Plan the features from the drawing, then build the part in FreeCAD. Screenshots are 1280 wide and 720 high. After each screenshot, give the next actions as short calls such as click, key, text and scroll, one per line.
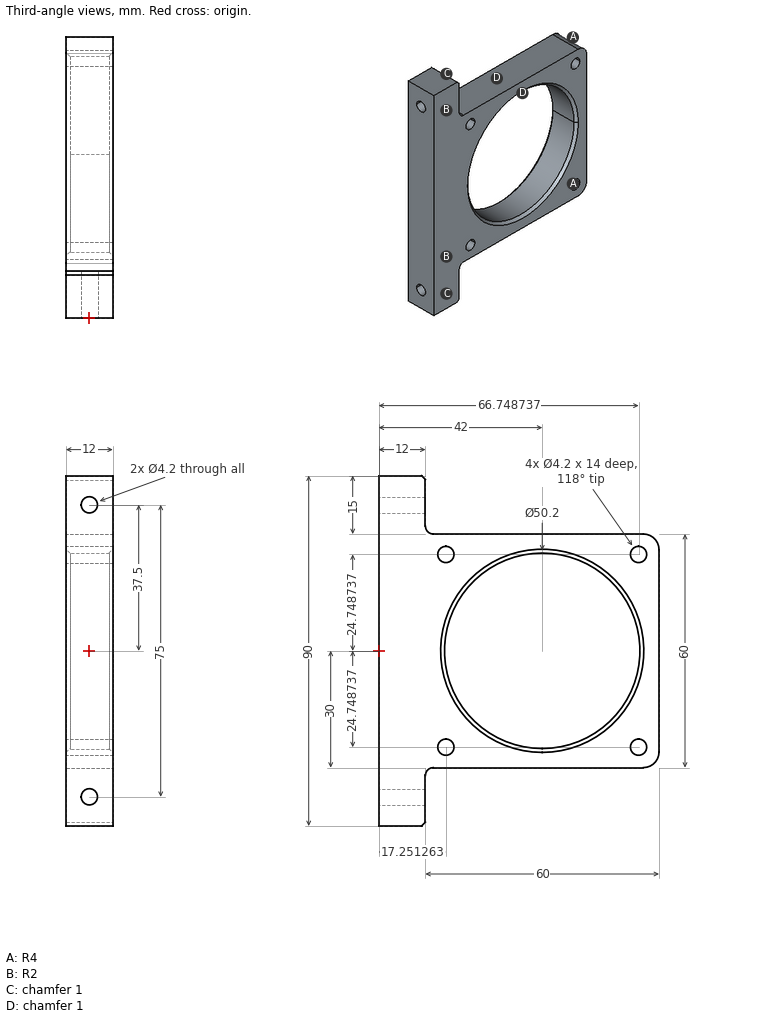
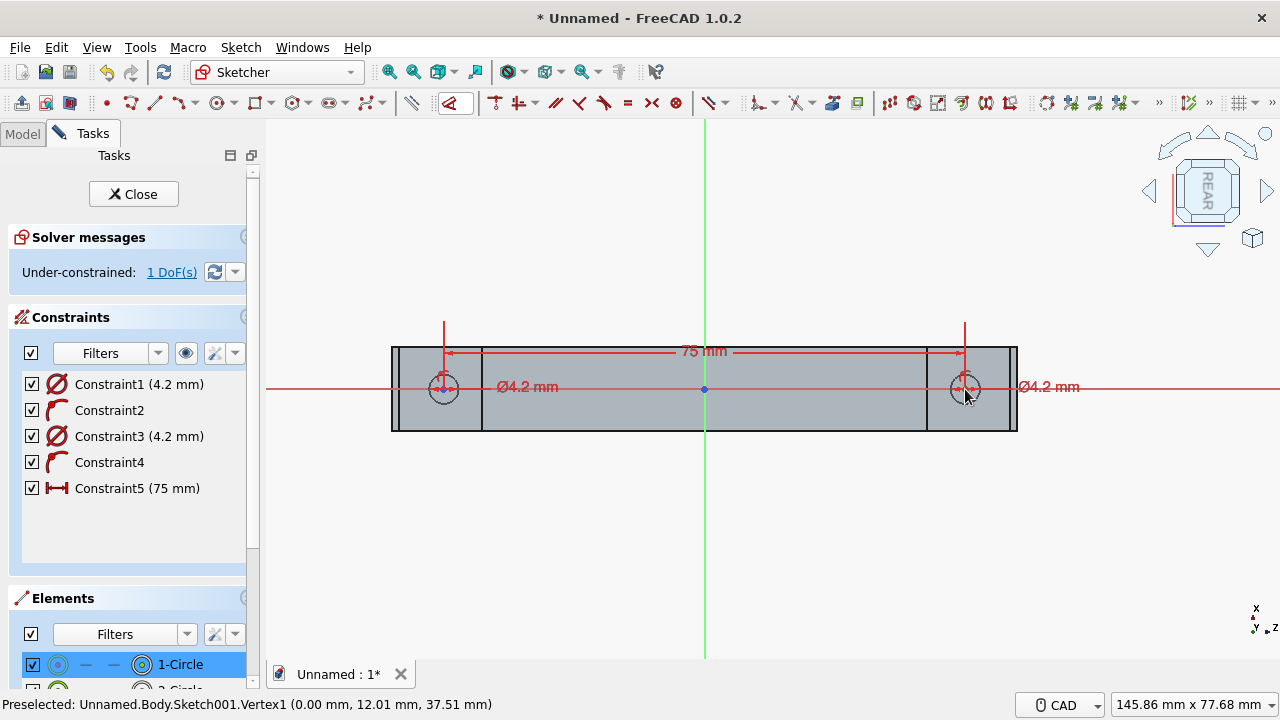
key(l)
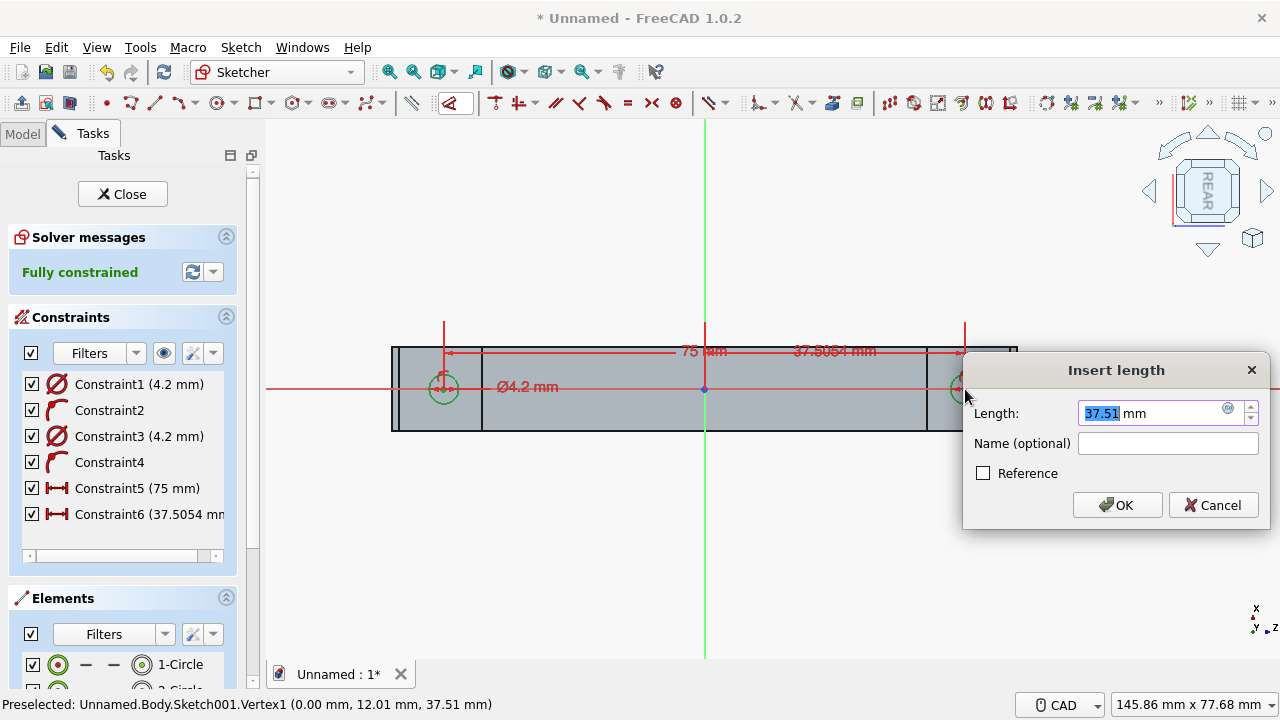
text(37.5)
key(Return)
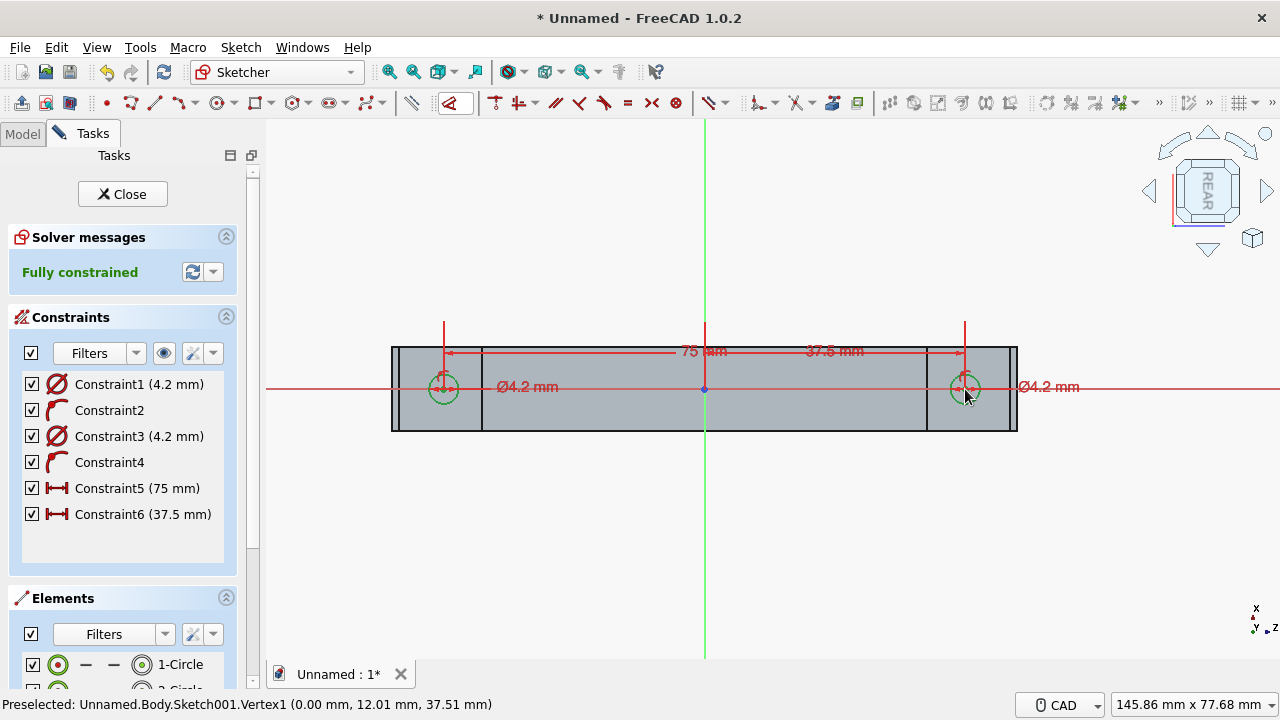
click(123, 194)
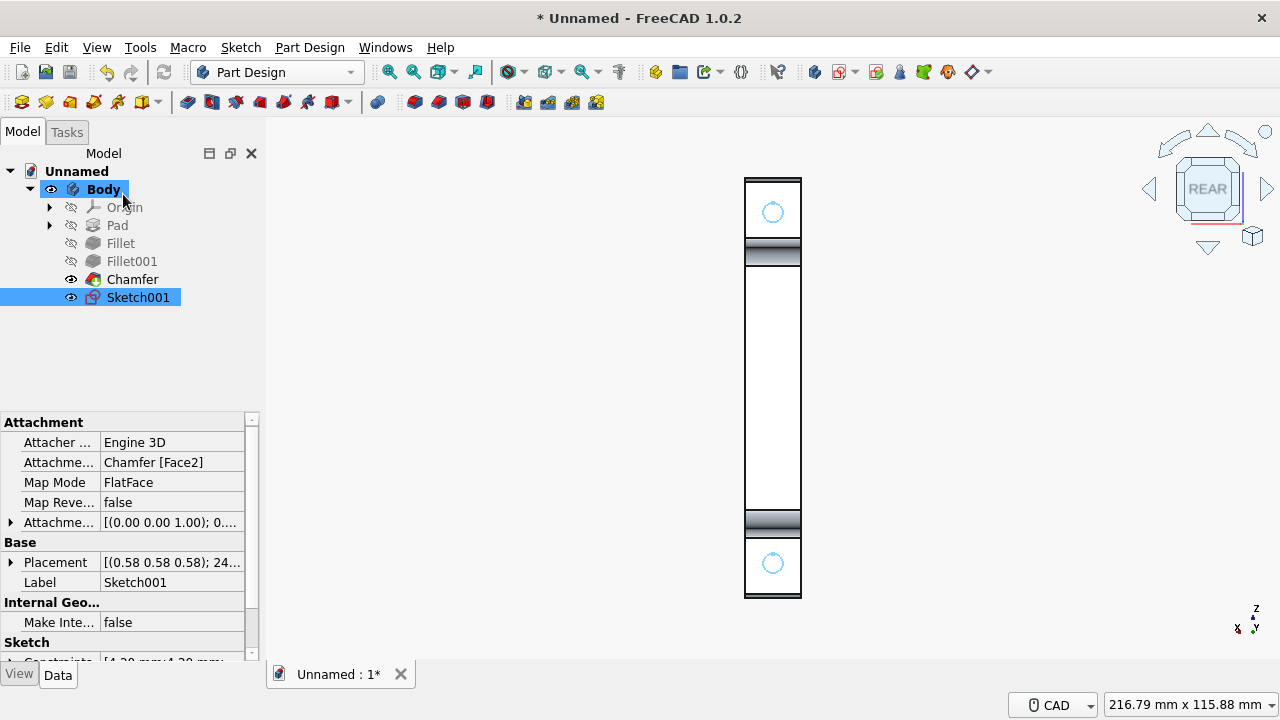
click(212, 102)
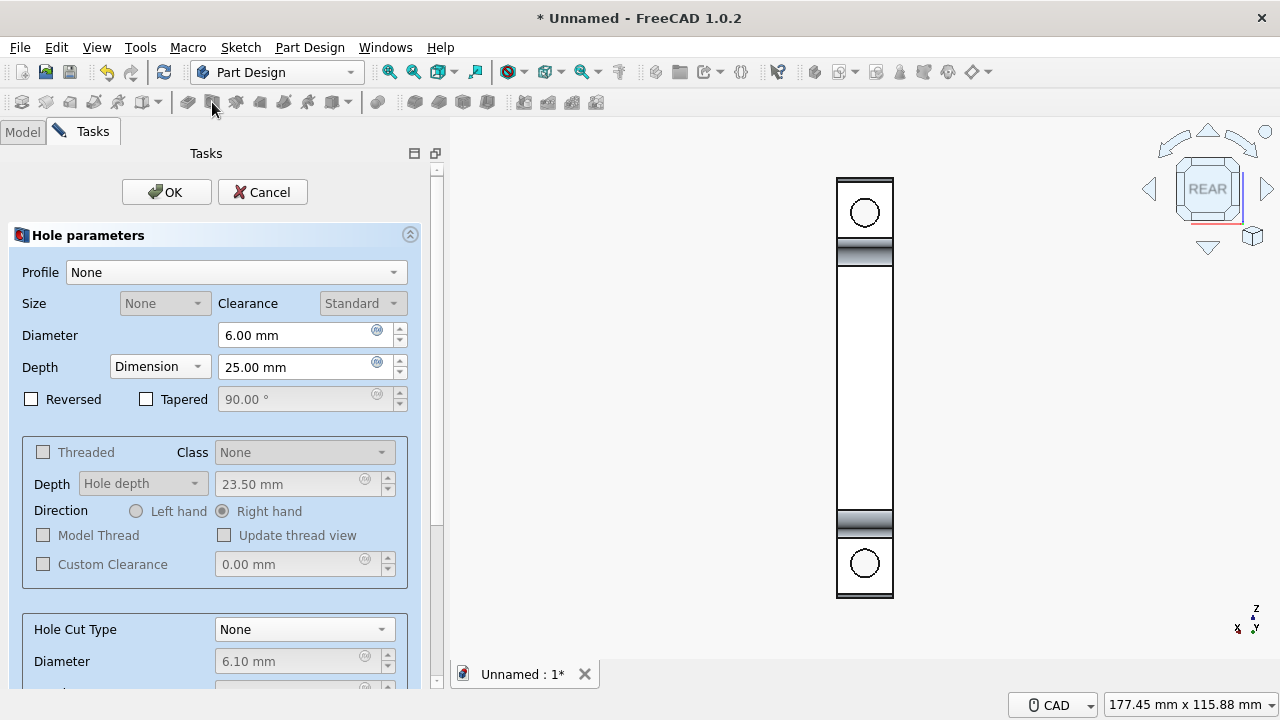
triple_click(305, 335)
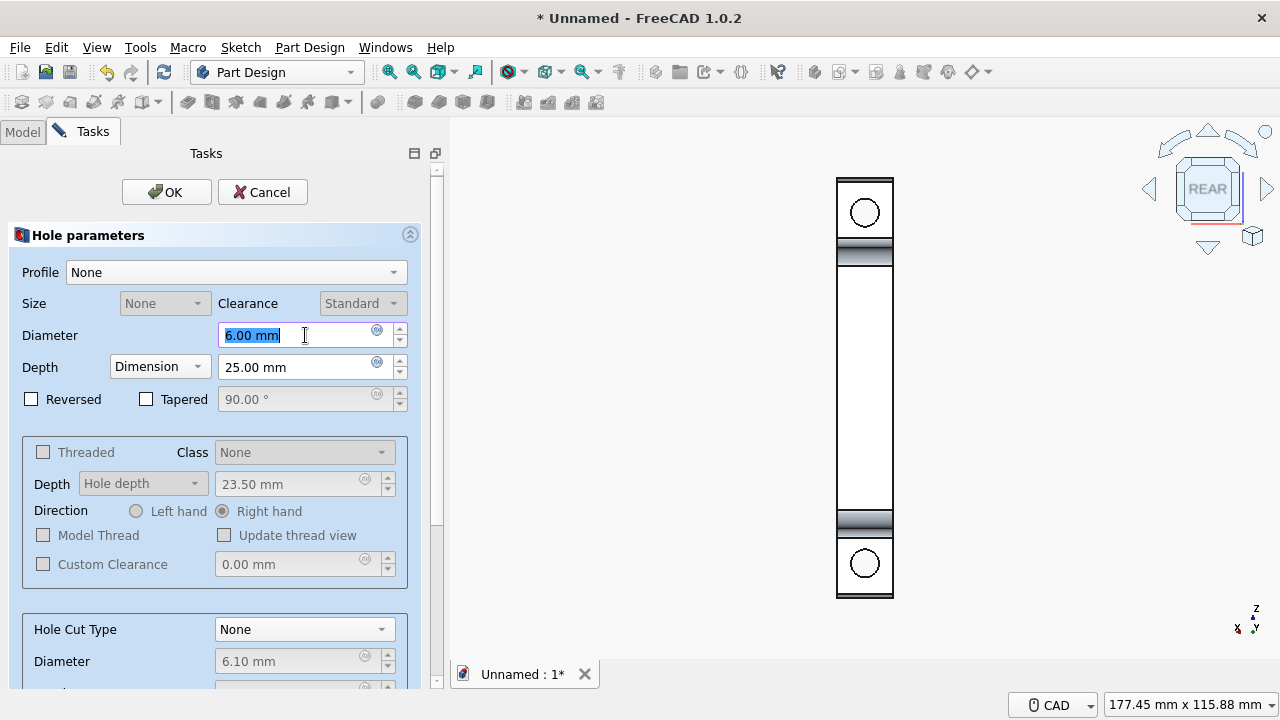
text(4.2)
key(Tab)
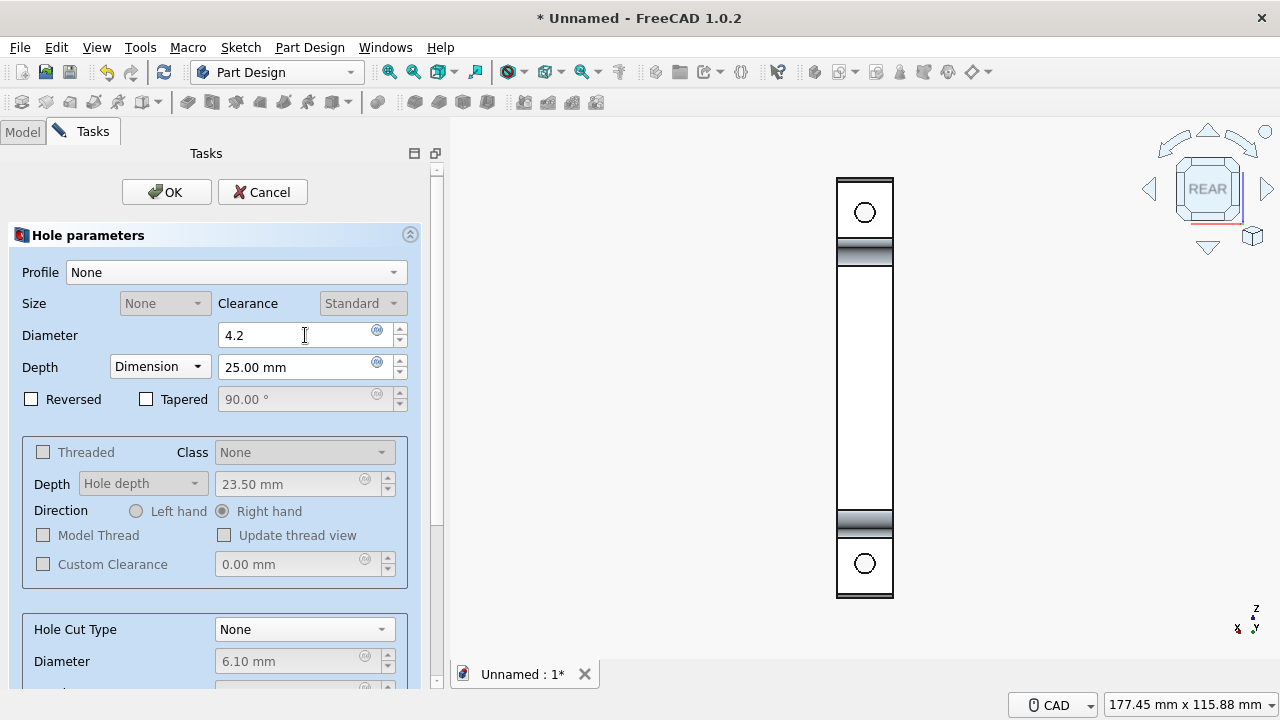
click(161, 366)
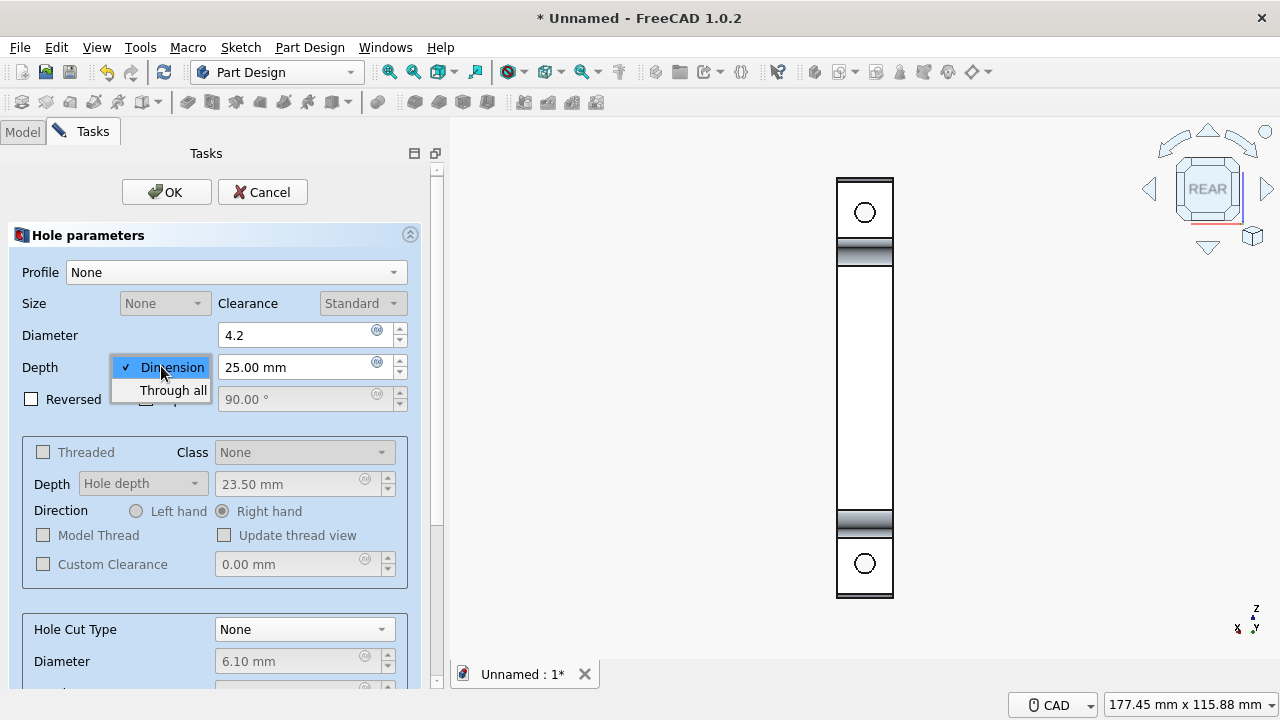
click(160, 390)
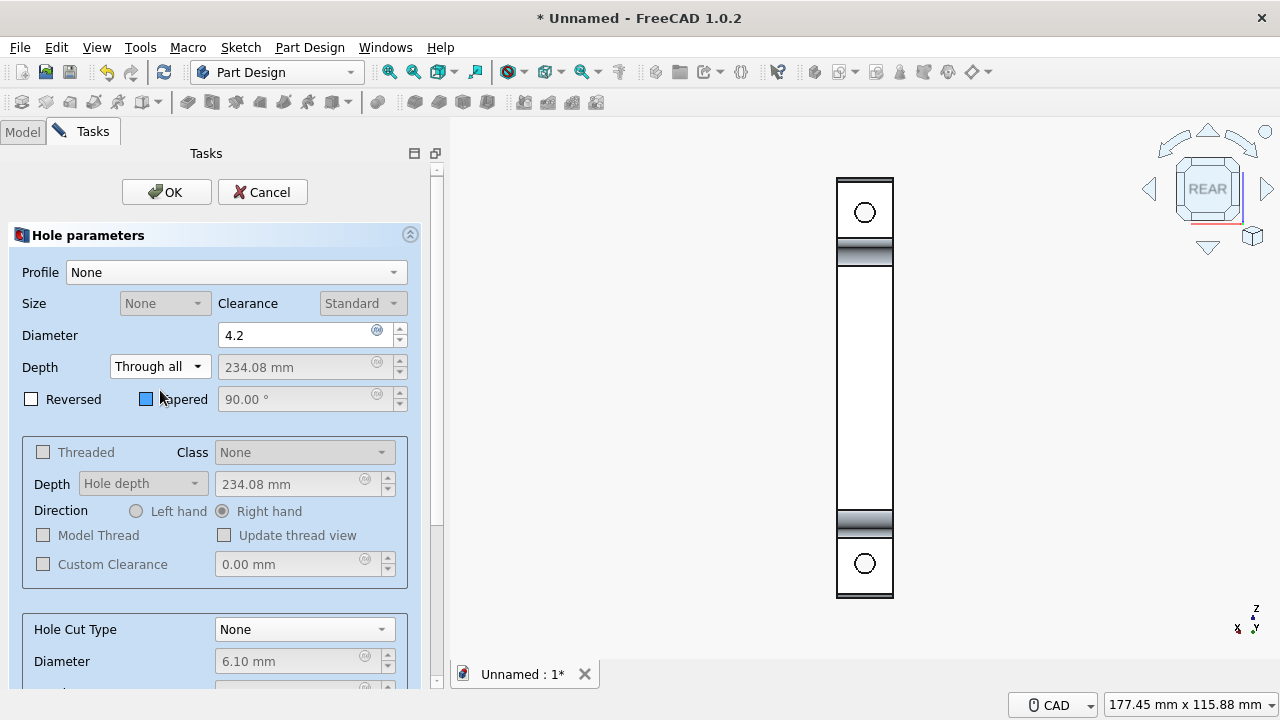
click(167, 192)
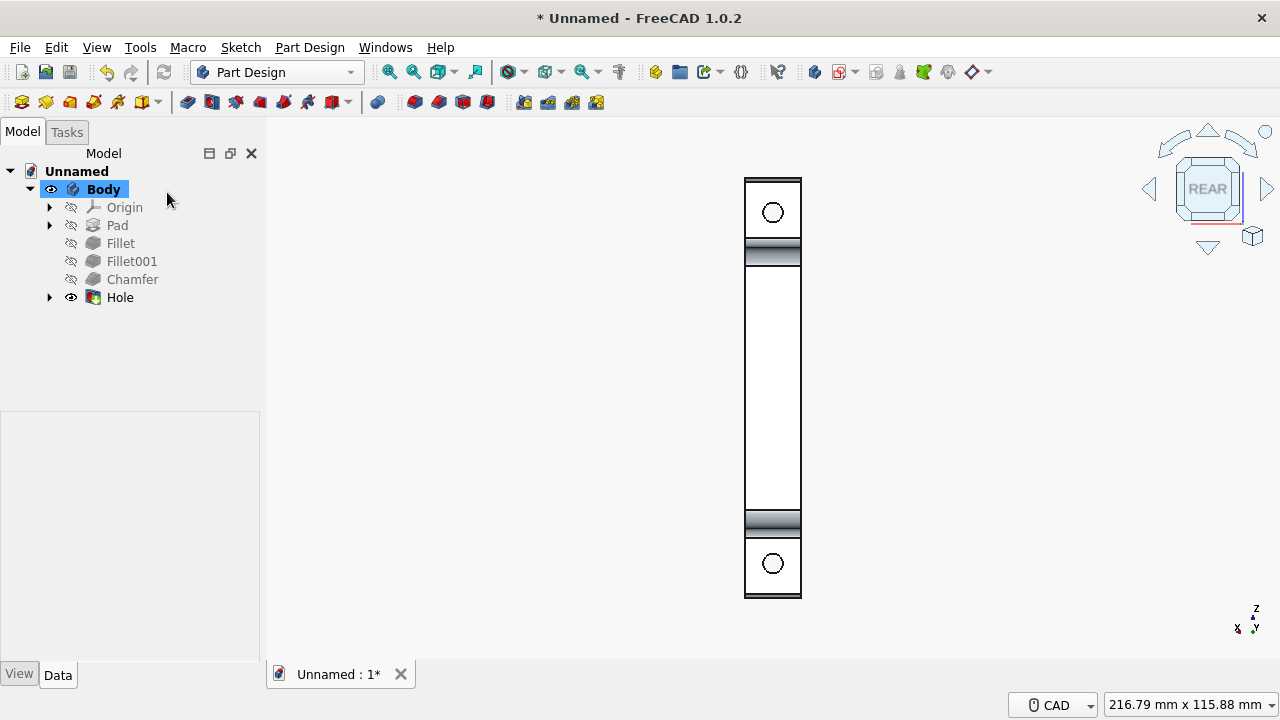
key(0)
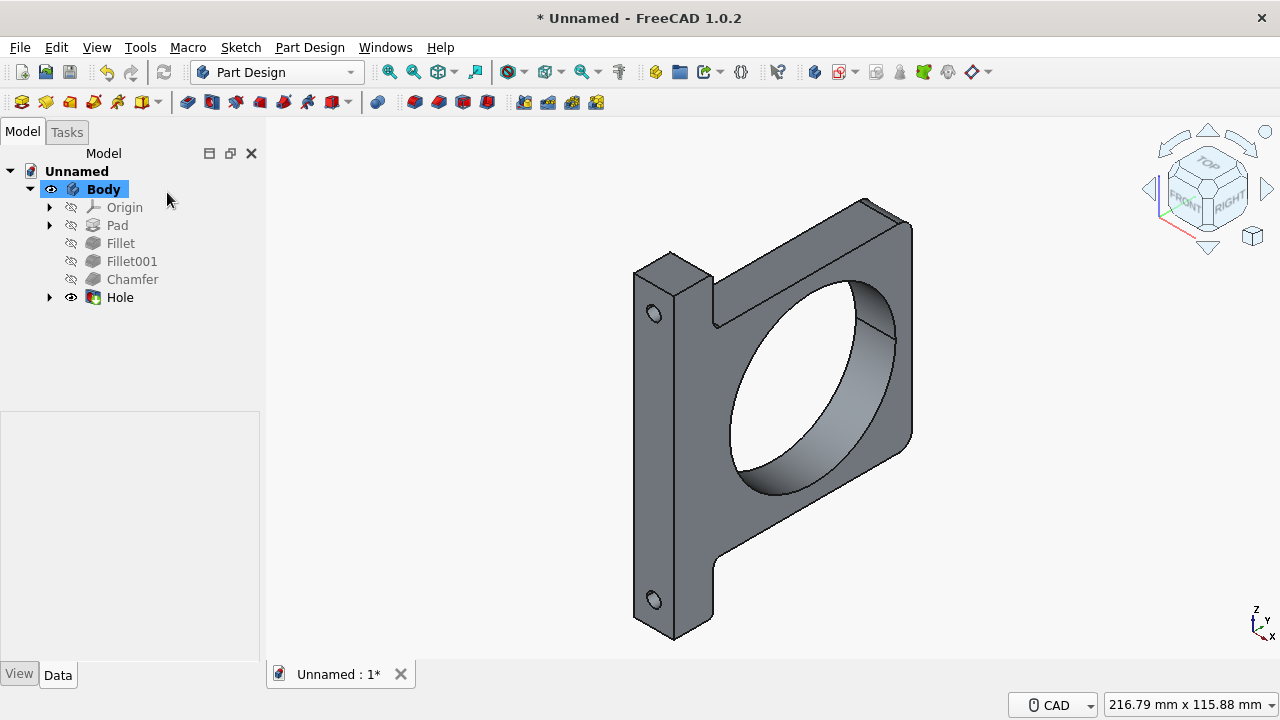
click(691, 605)